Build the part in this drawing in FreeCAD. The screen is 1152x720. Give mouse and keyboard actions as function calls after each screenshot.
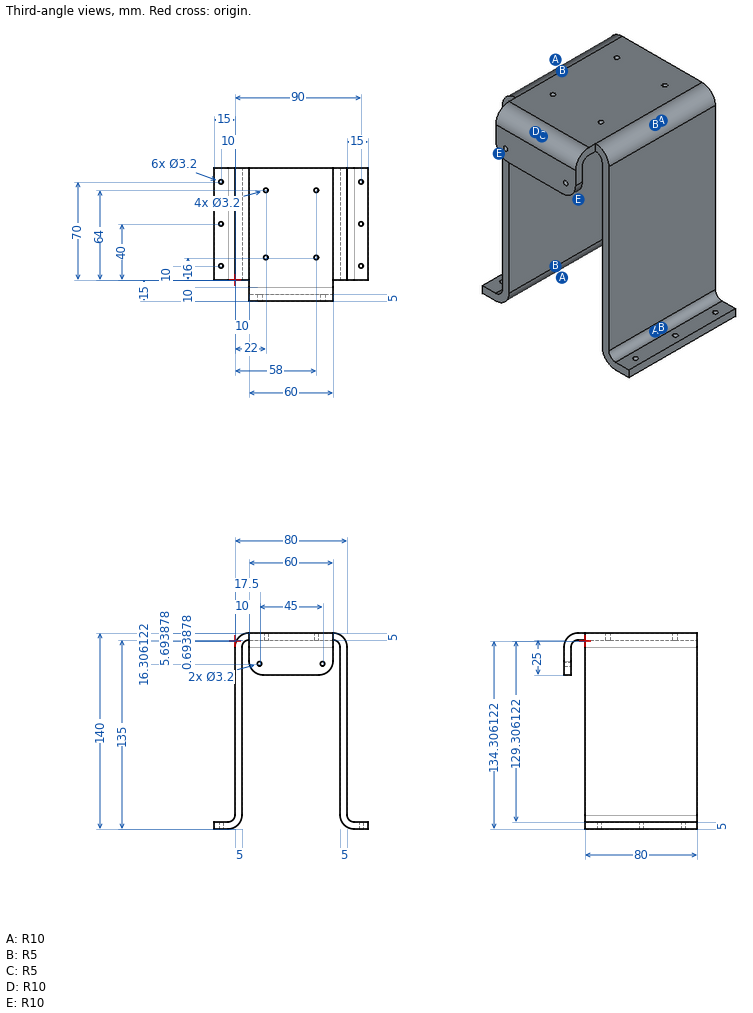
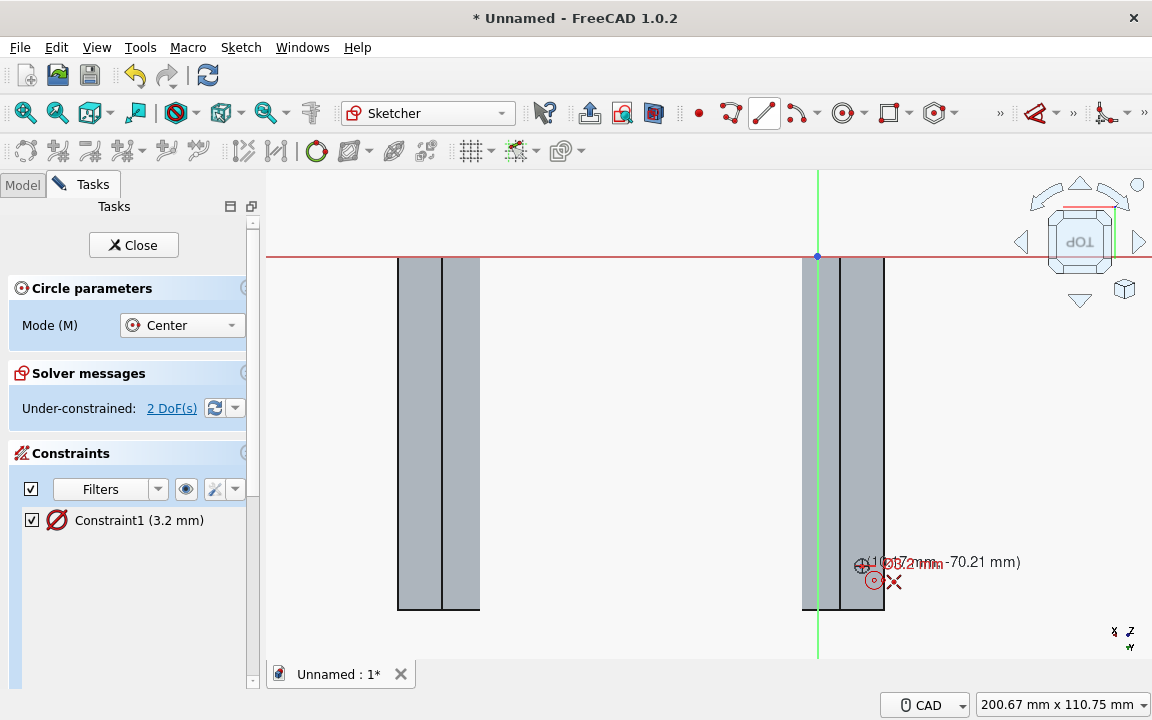
scroll(862, 433, up, 6)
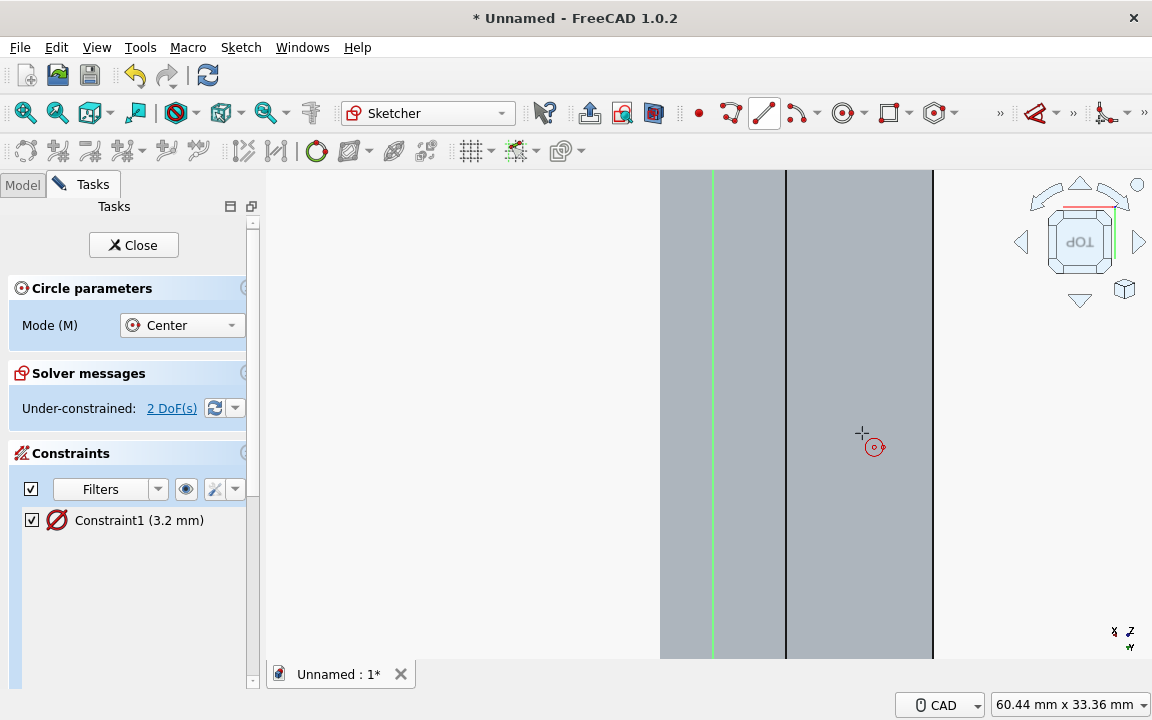
click(860, 433)
move(876, 417)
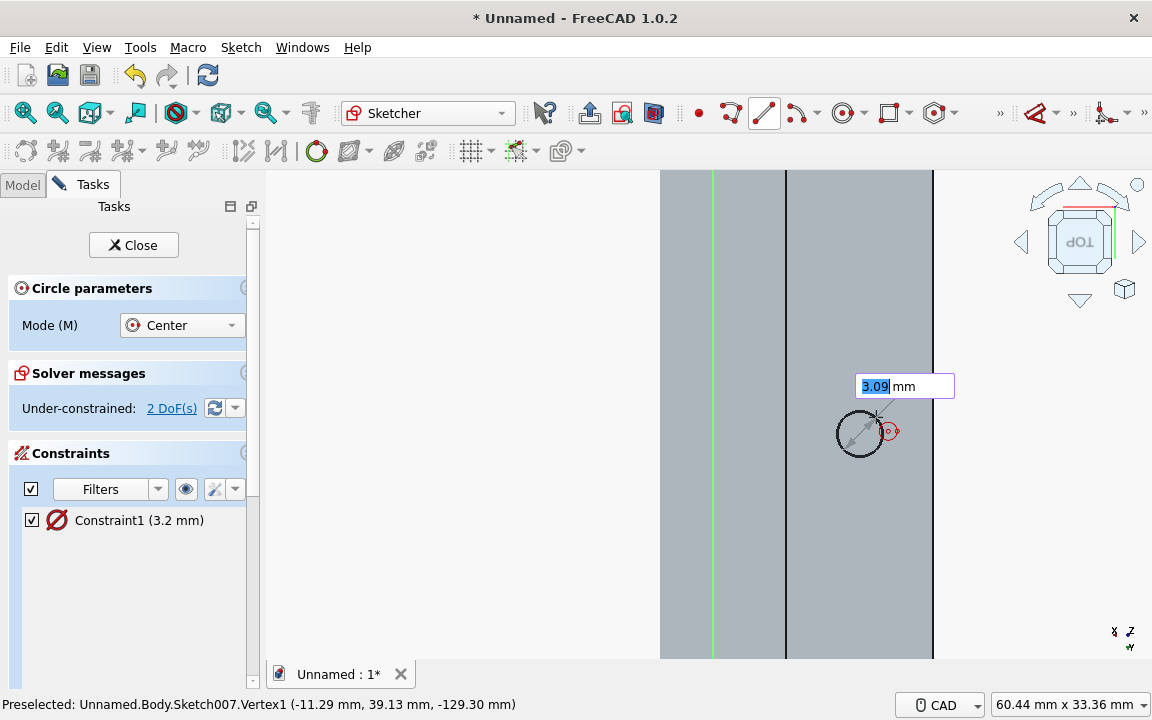
text(3.2)
key(Return)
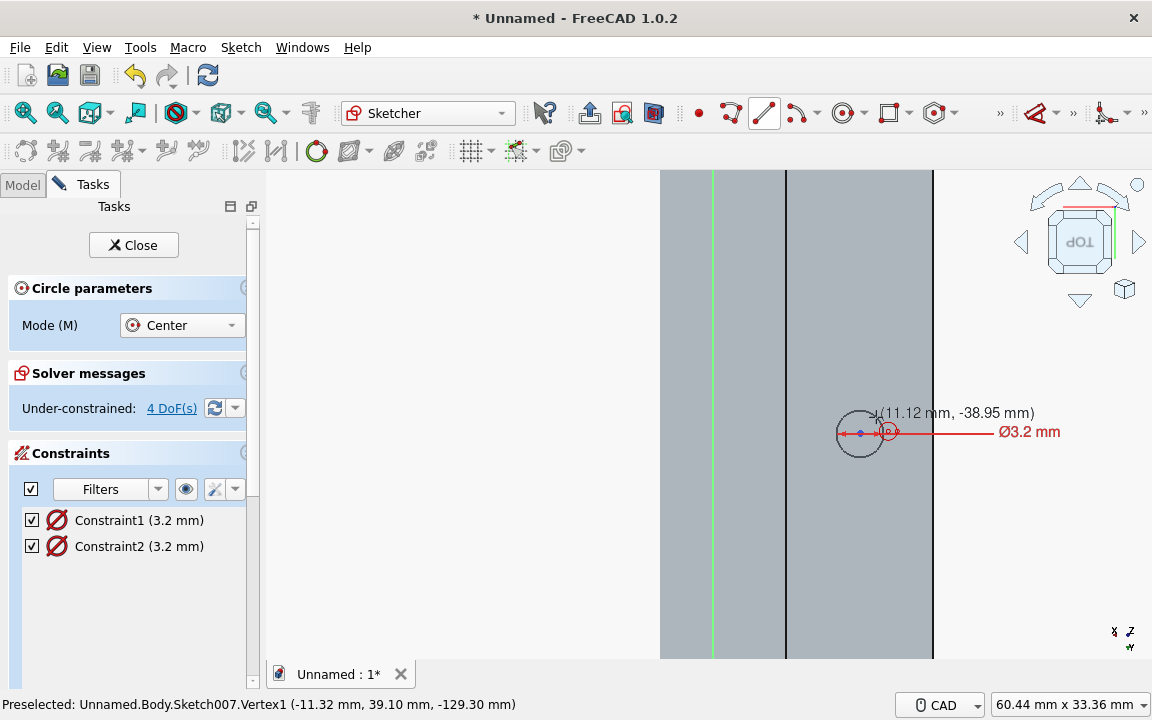
scroll(862, 433, down, 6)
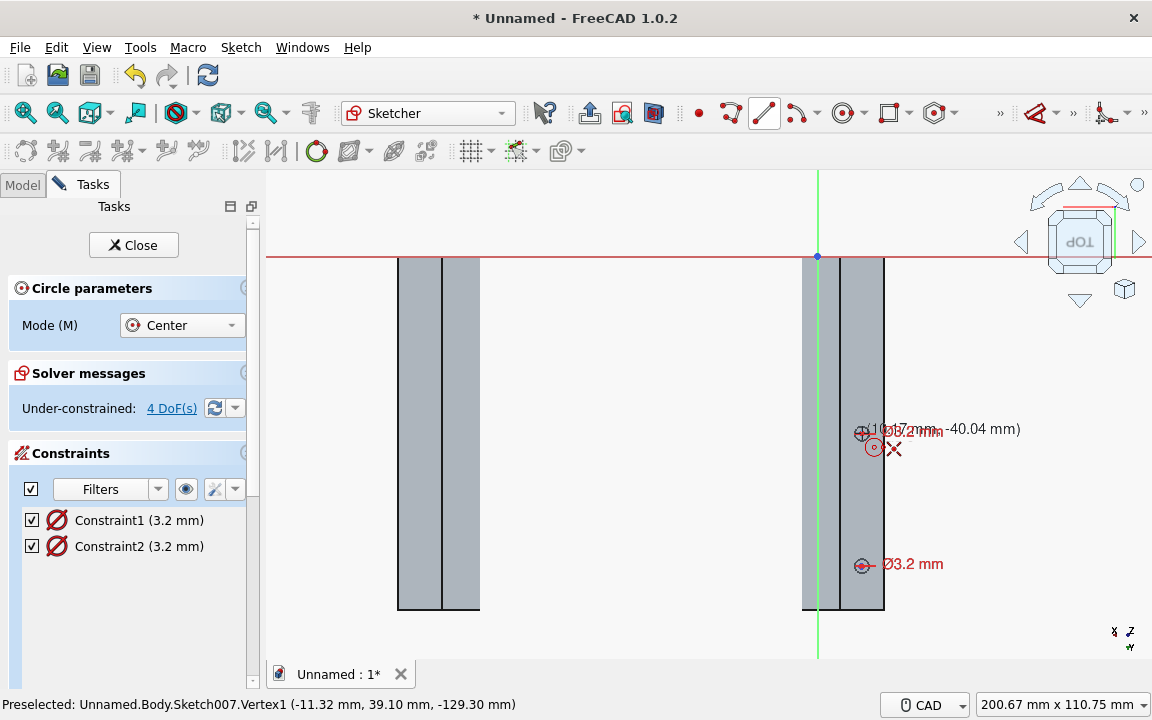
scroll(862, 301, up, 6)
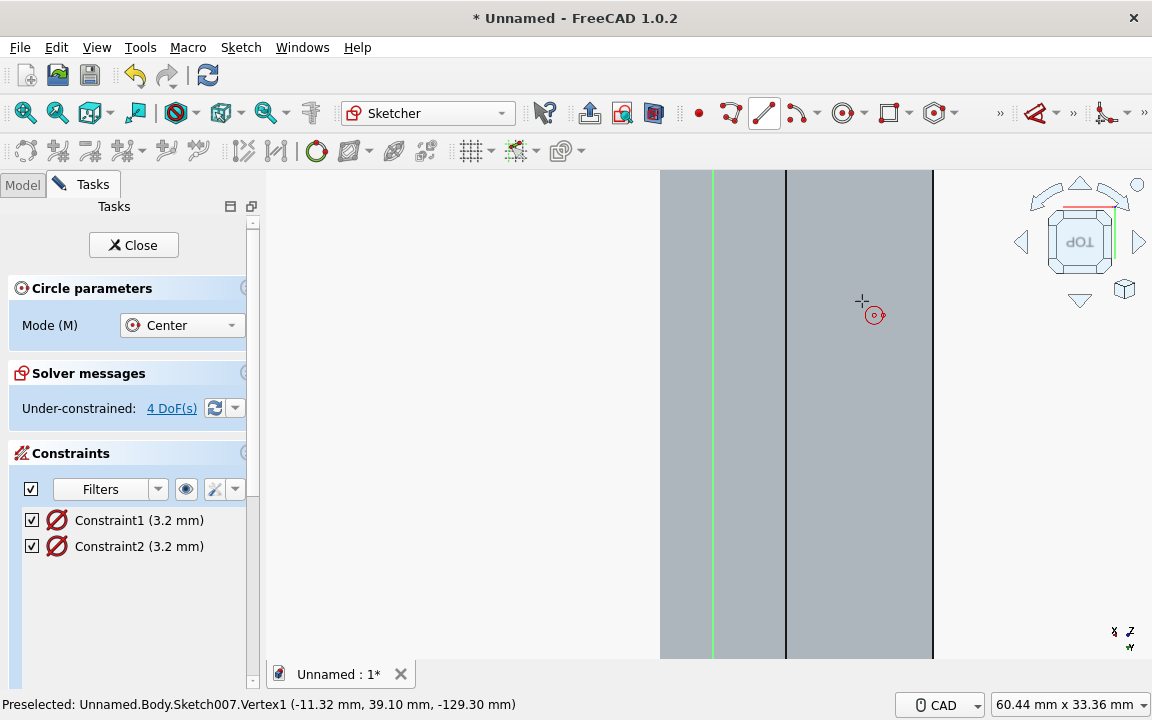
click(860, 300)
move(876, 284)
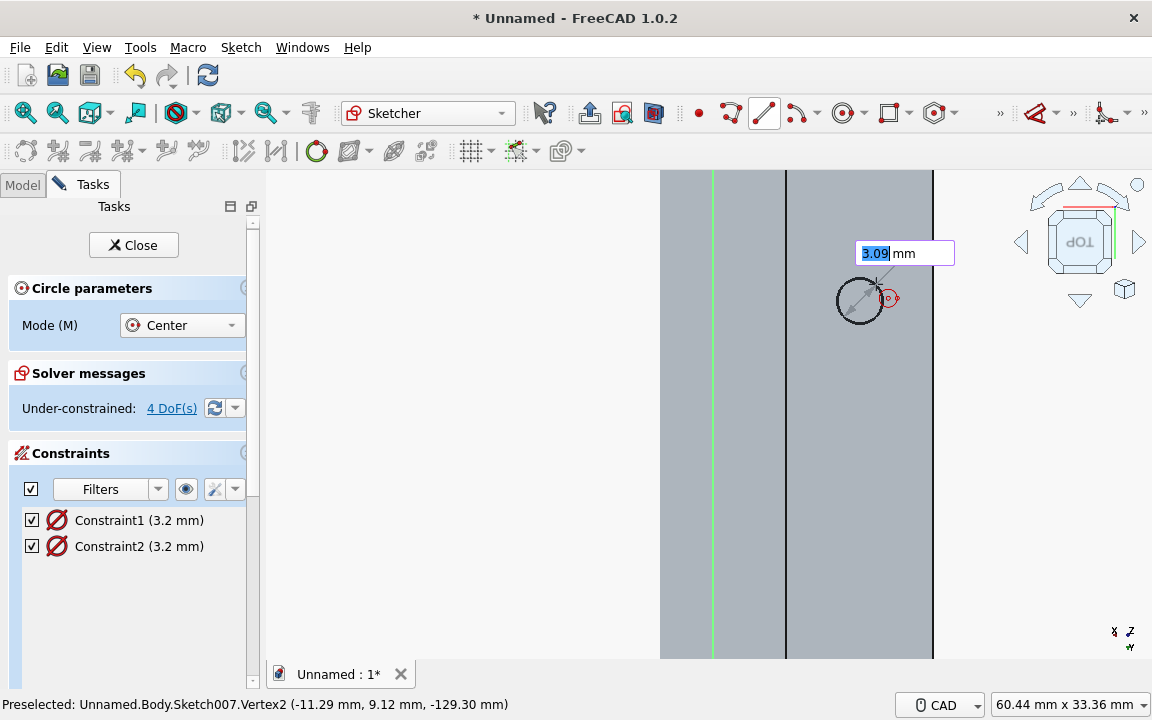
text(3.2)
key(Return)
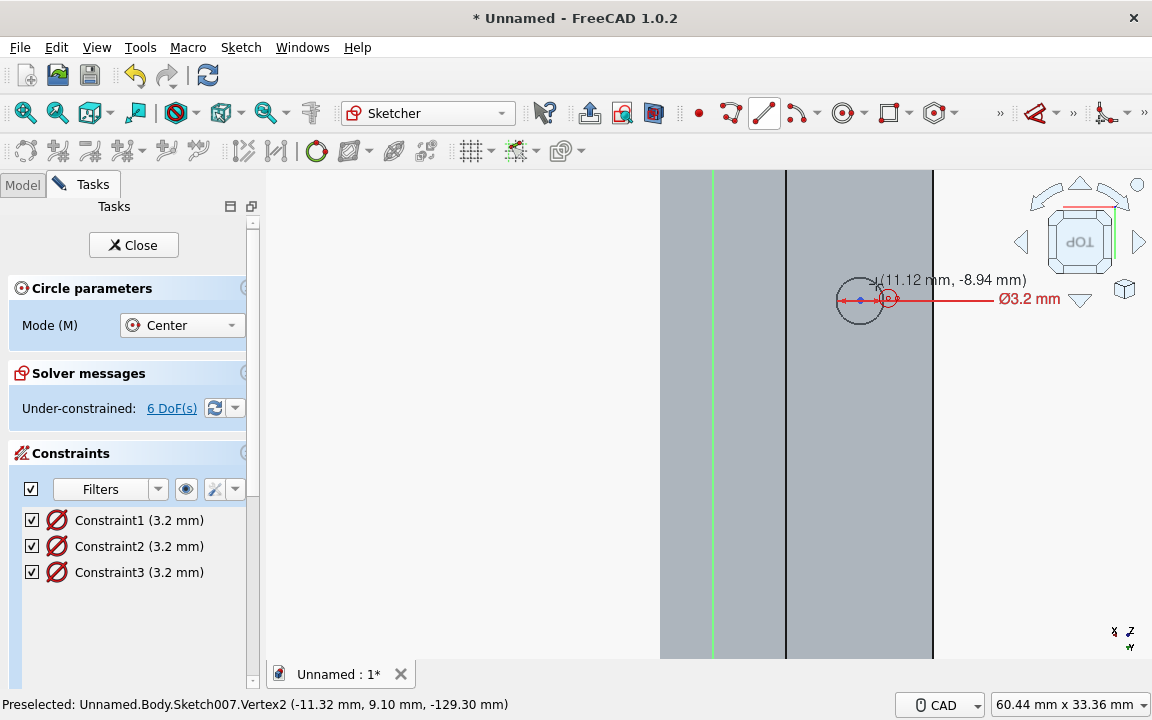
scroll(862, 301, down, 6)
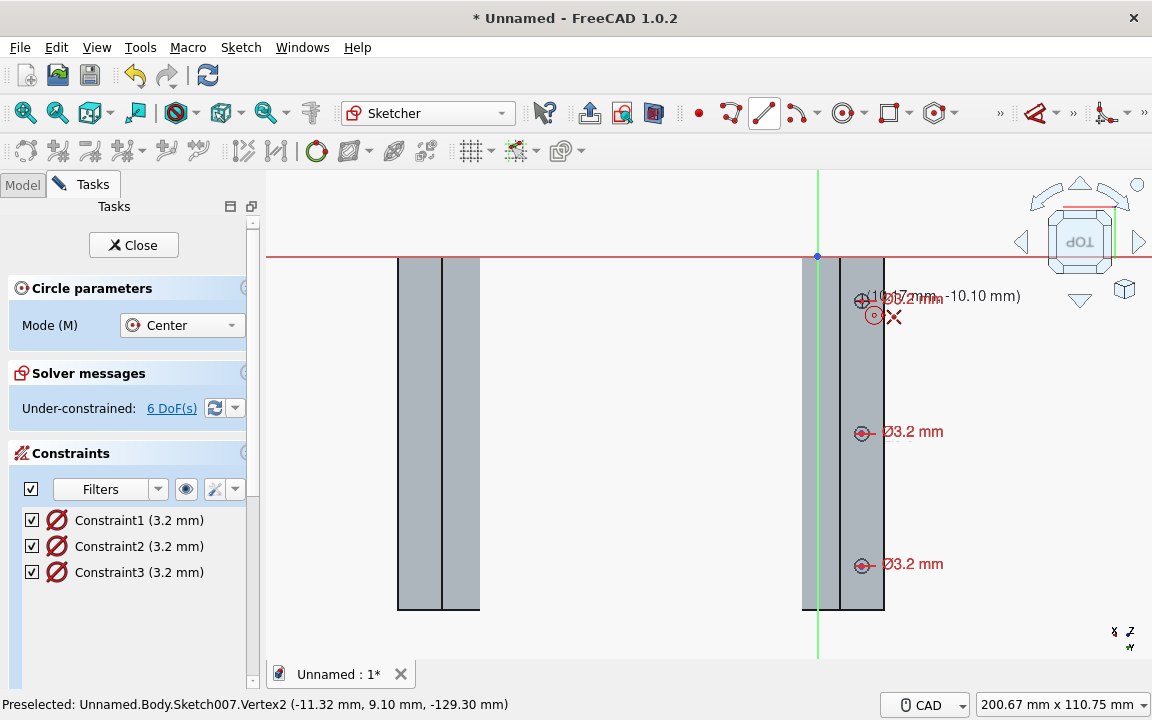
scroll(420, 566, up, 6)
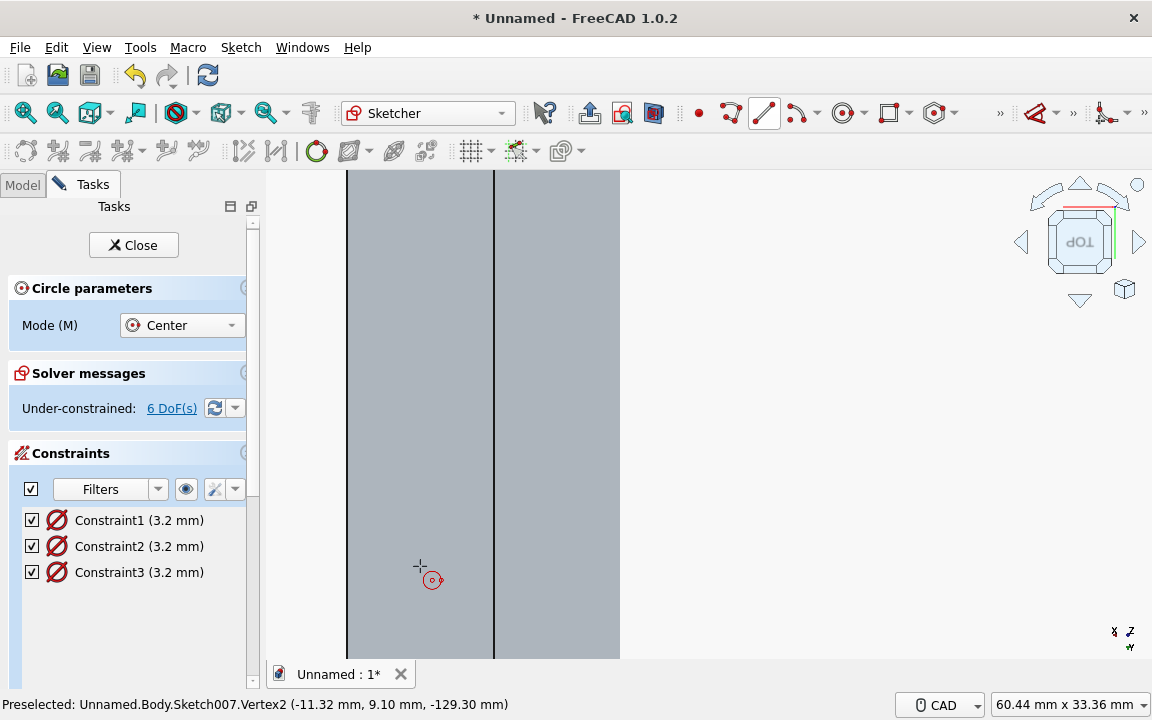
click(420, 564)
move(437, 547)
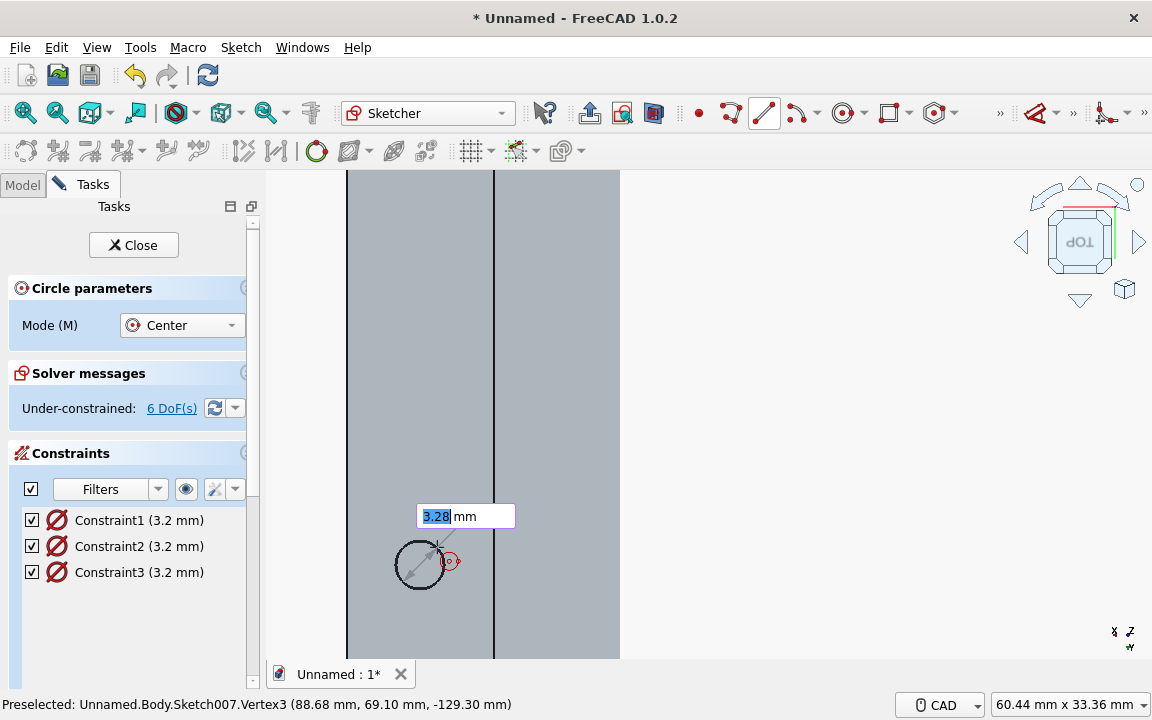
text(3.2)
key(Return)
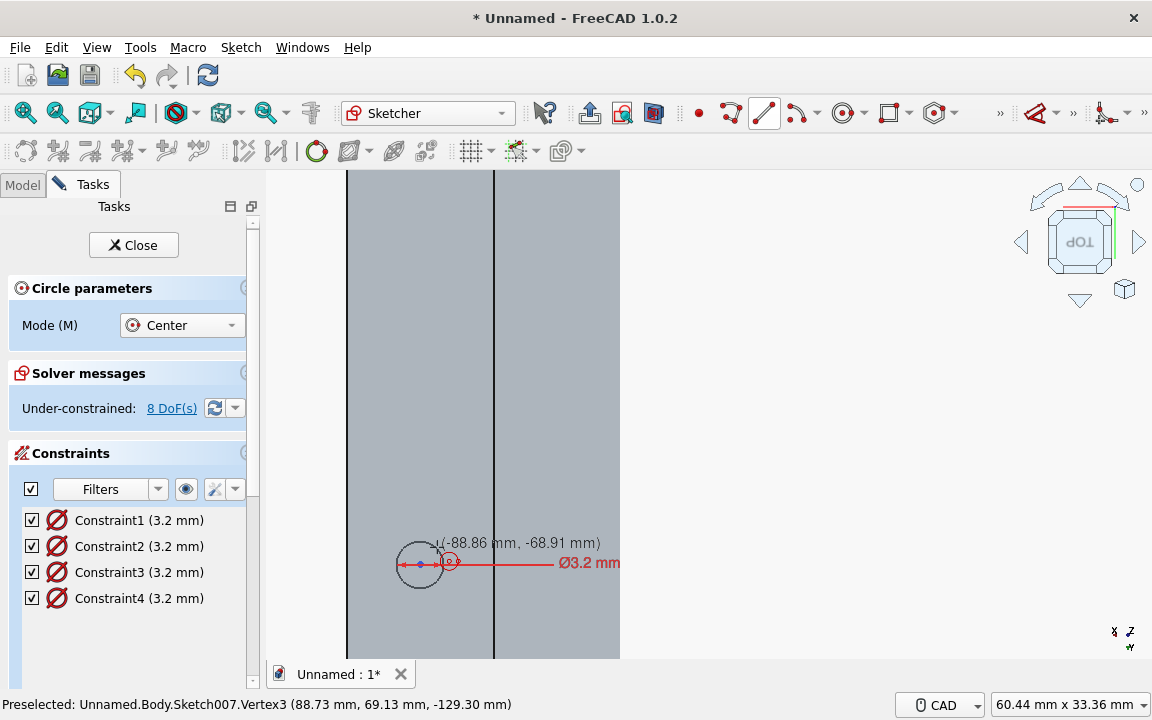
scroll(419, 566, down, 6)